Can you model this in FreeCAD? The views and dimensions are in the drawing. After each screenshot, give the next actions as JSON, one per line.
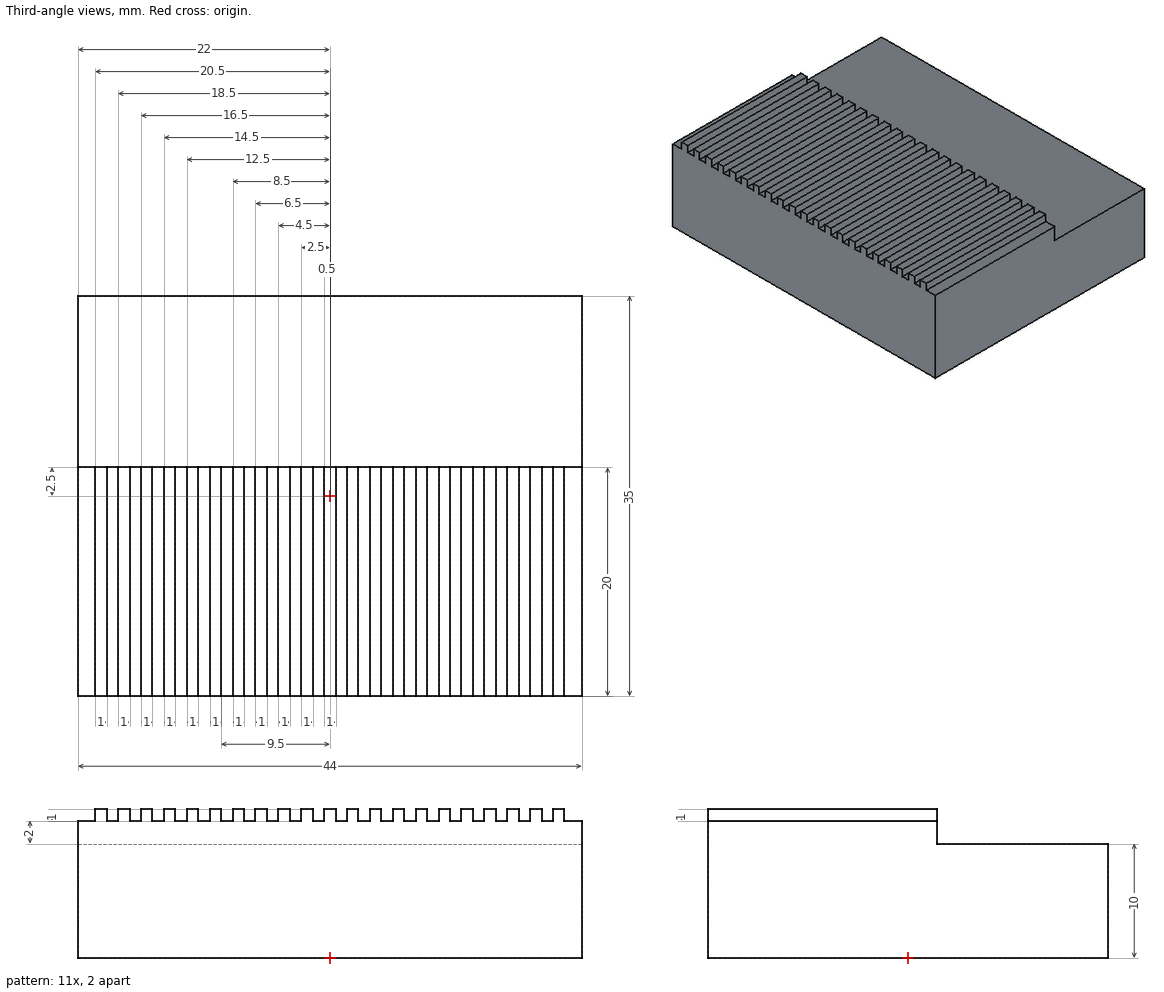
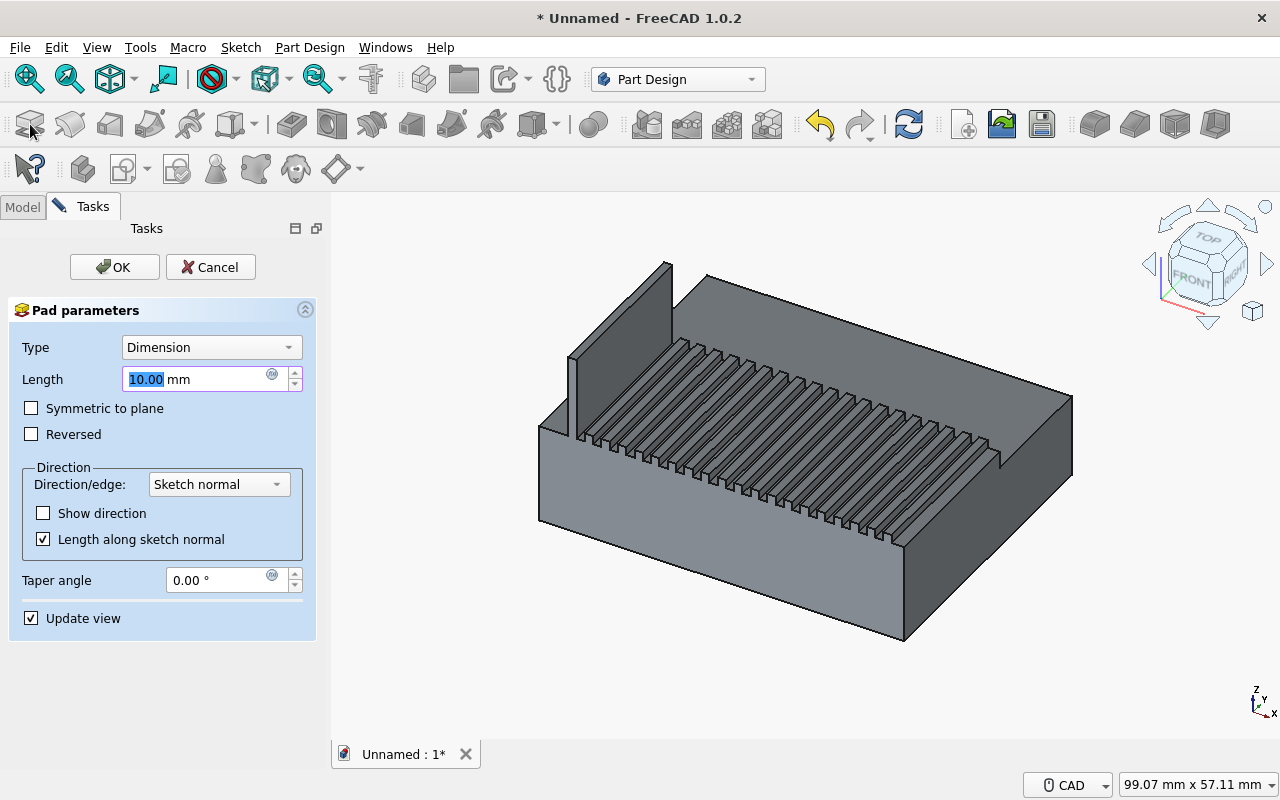
{"action": "type", "text": "1"}
{"action": "key", "text": "Tab"}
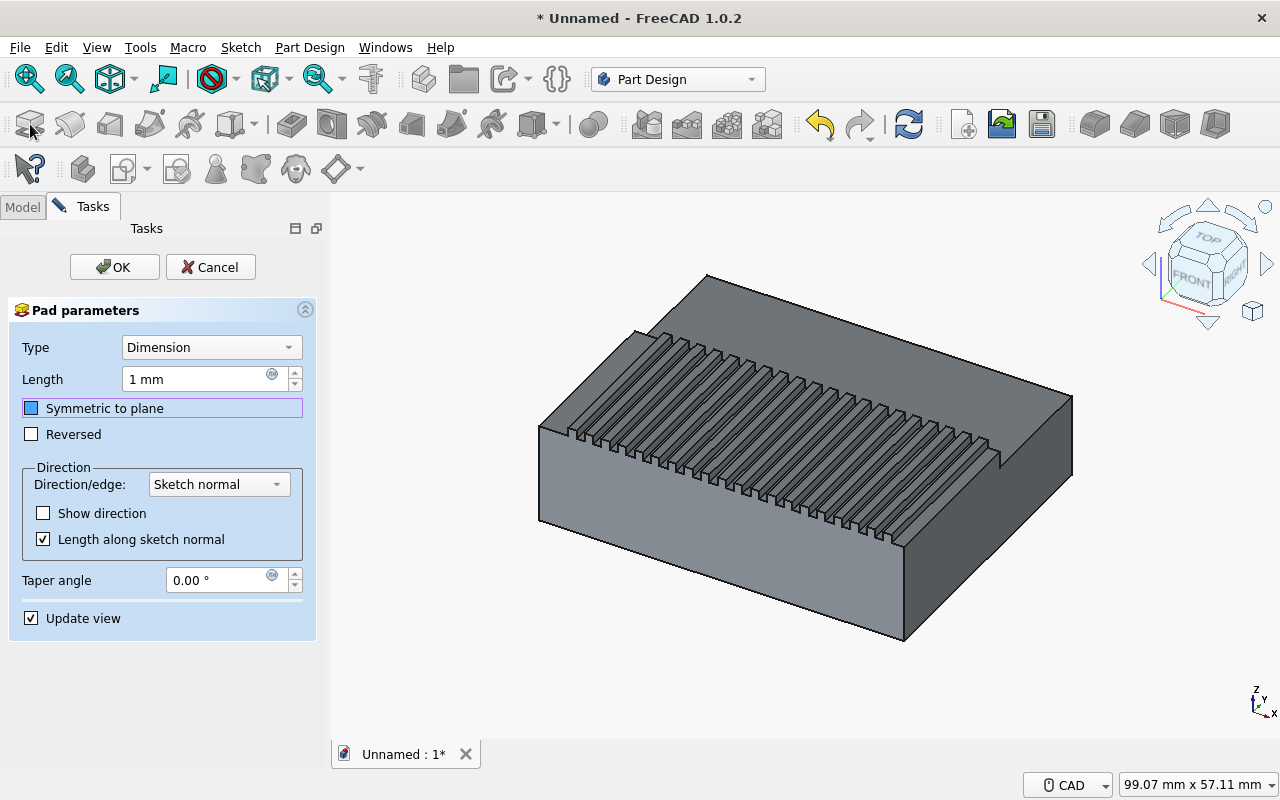
{"action": "left_click", "coordinate": [115, 267]}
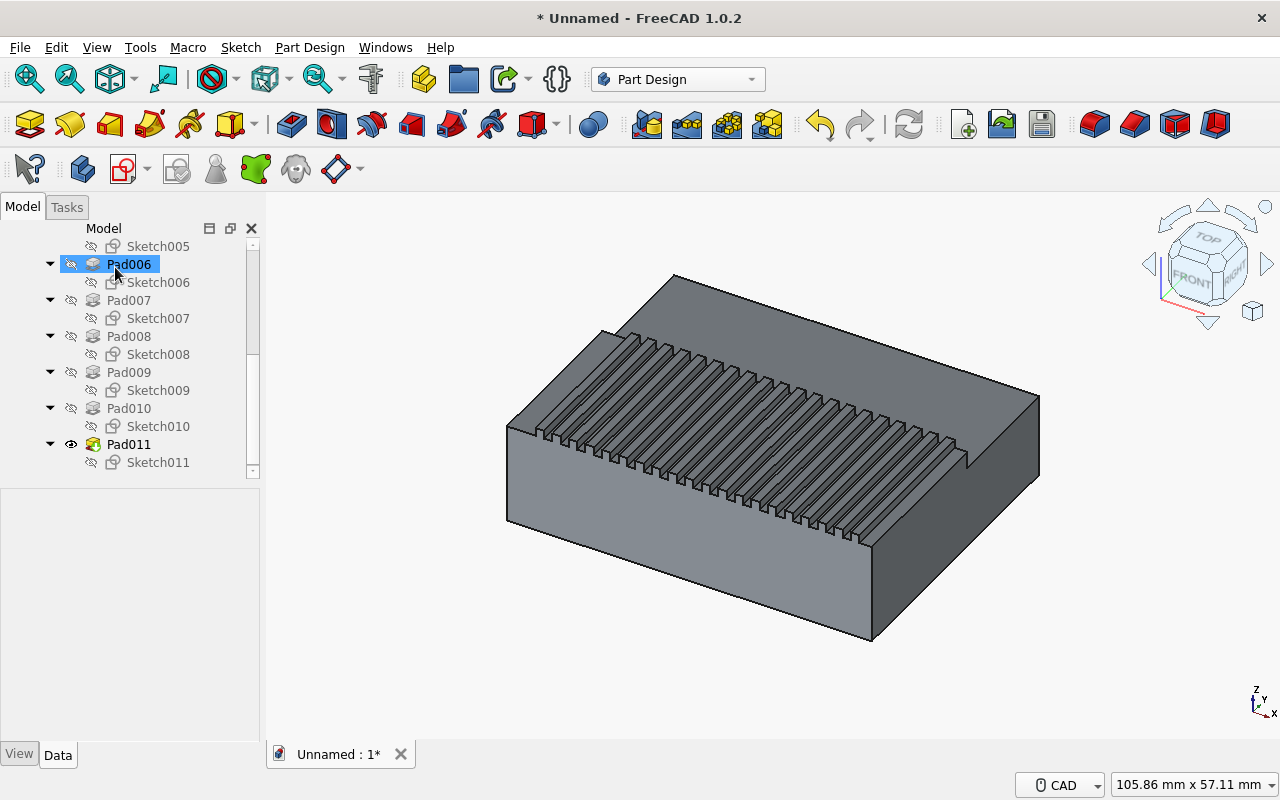
{"action": "key", "text": "0"}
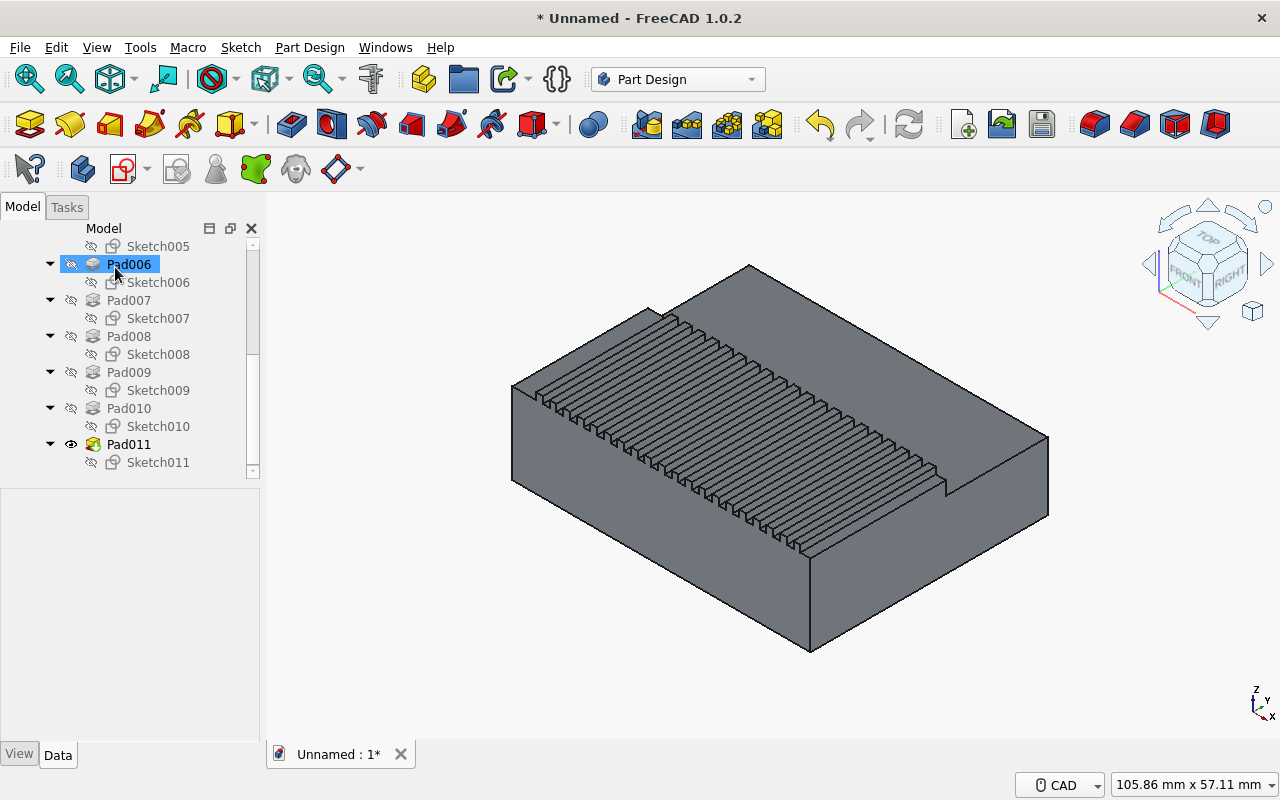
{"action": "key", "text": "2"}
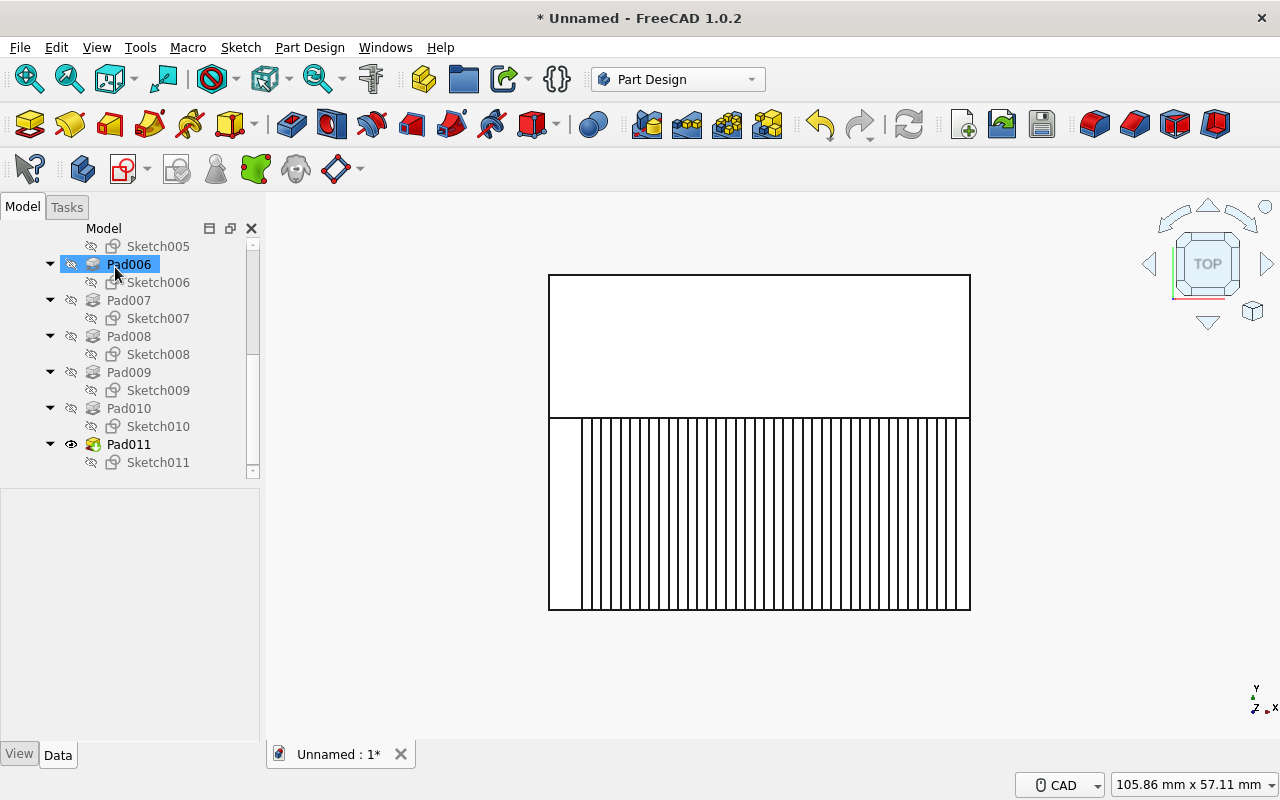
{"action": "left_click", "coordinate": [566, 458]}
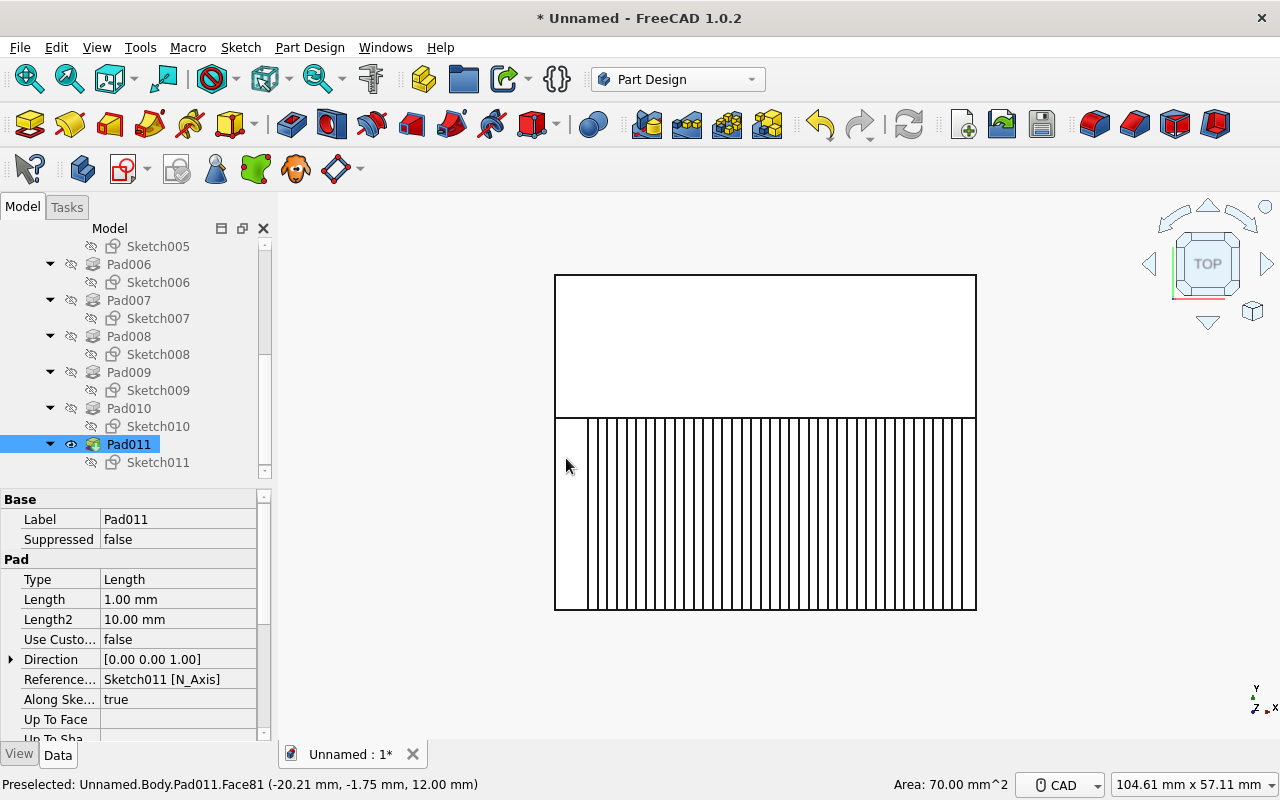
{"action": "left_click", "coordinate": [124, 170]}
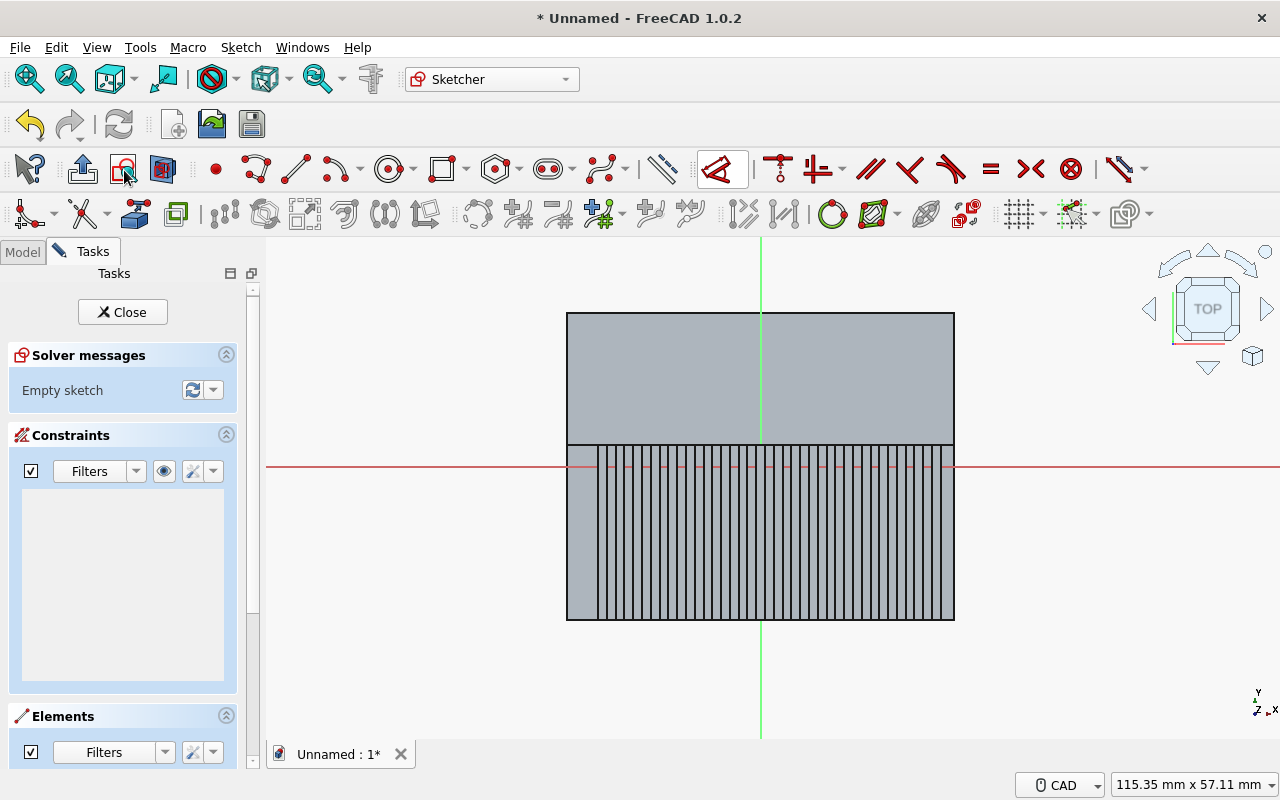
{"action": "scroll", "coordinate": [629, 587], "scroll_direction": "up", "scroll_amount": 3}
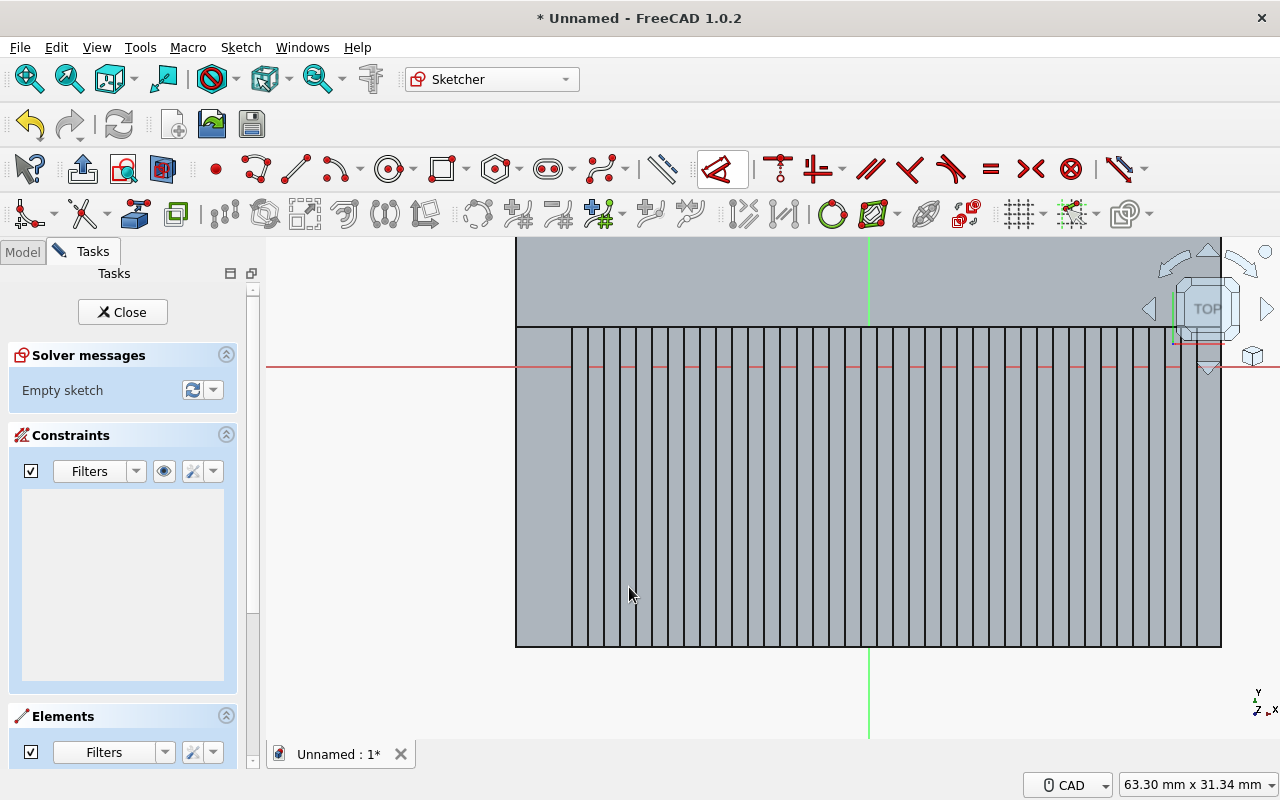
{"action": "left_click", "coordinate": [442, 170]}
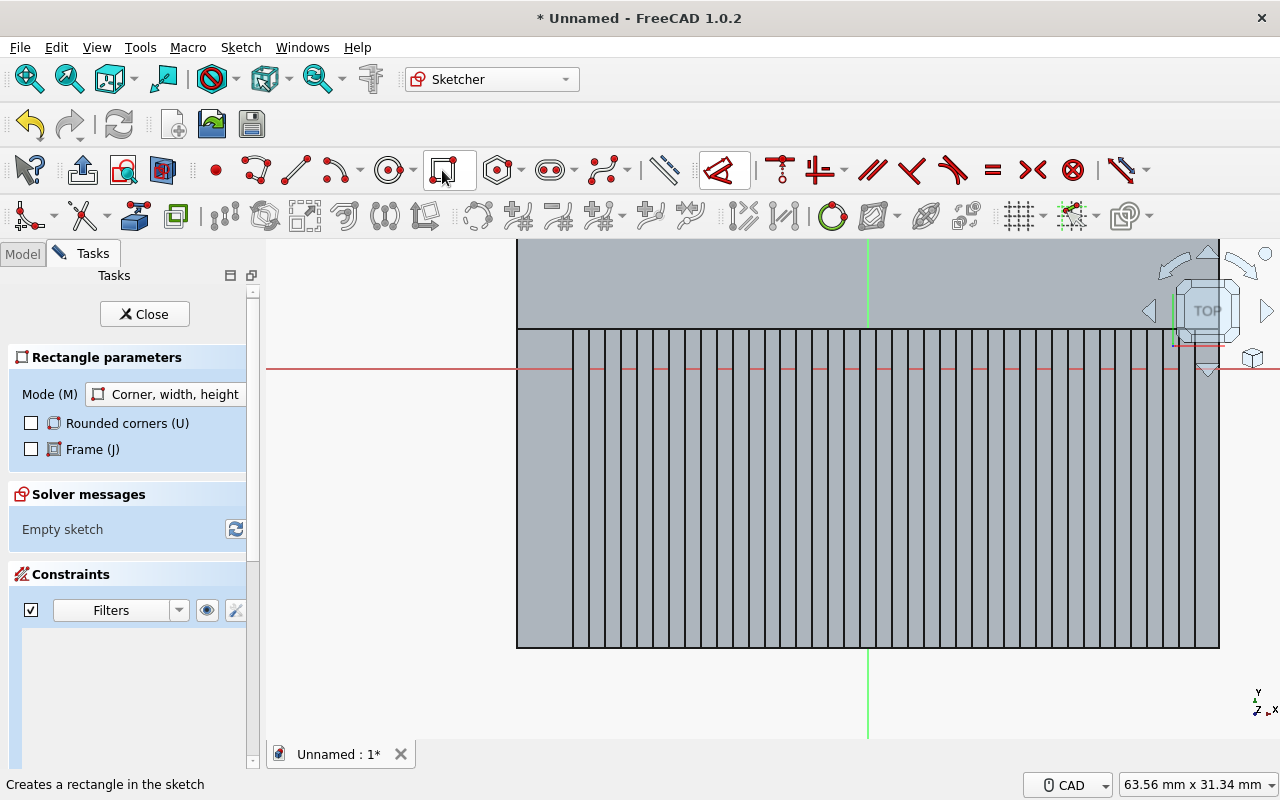
{"action": "left_click", "coordinate": [541, 329]}
{"action": "mouse_move", "coordinate": [557, 648]}